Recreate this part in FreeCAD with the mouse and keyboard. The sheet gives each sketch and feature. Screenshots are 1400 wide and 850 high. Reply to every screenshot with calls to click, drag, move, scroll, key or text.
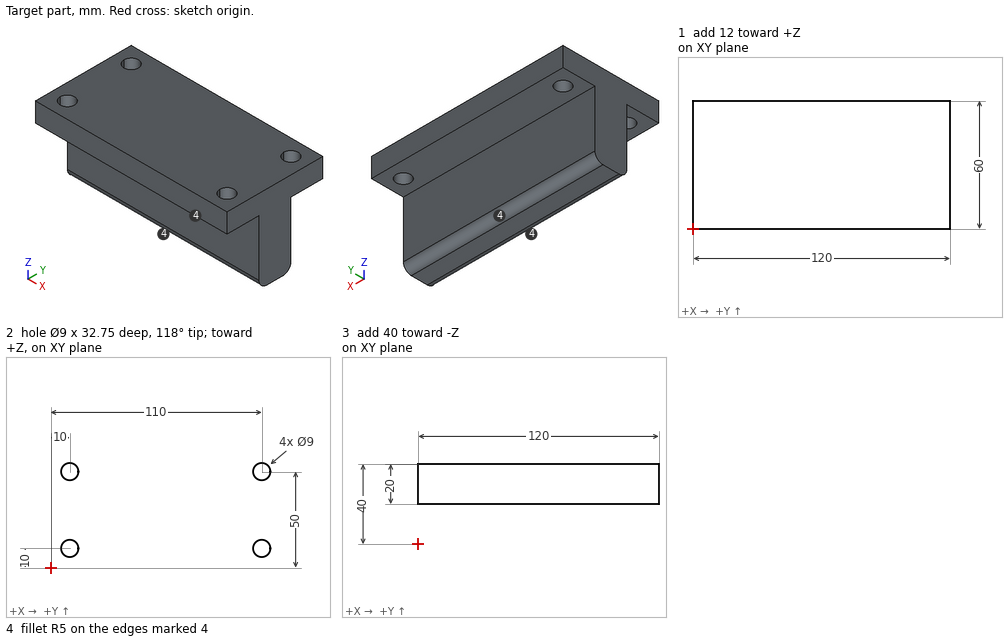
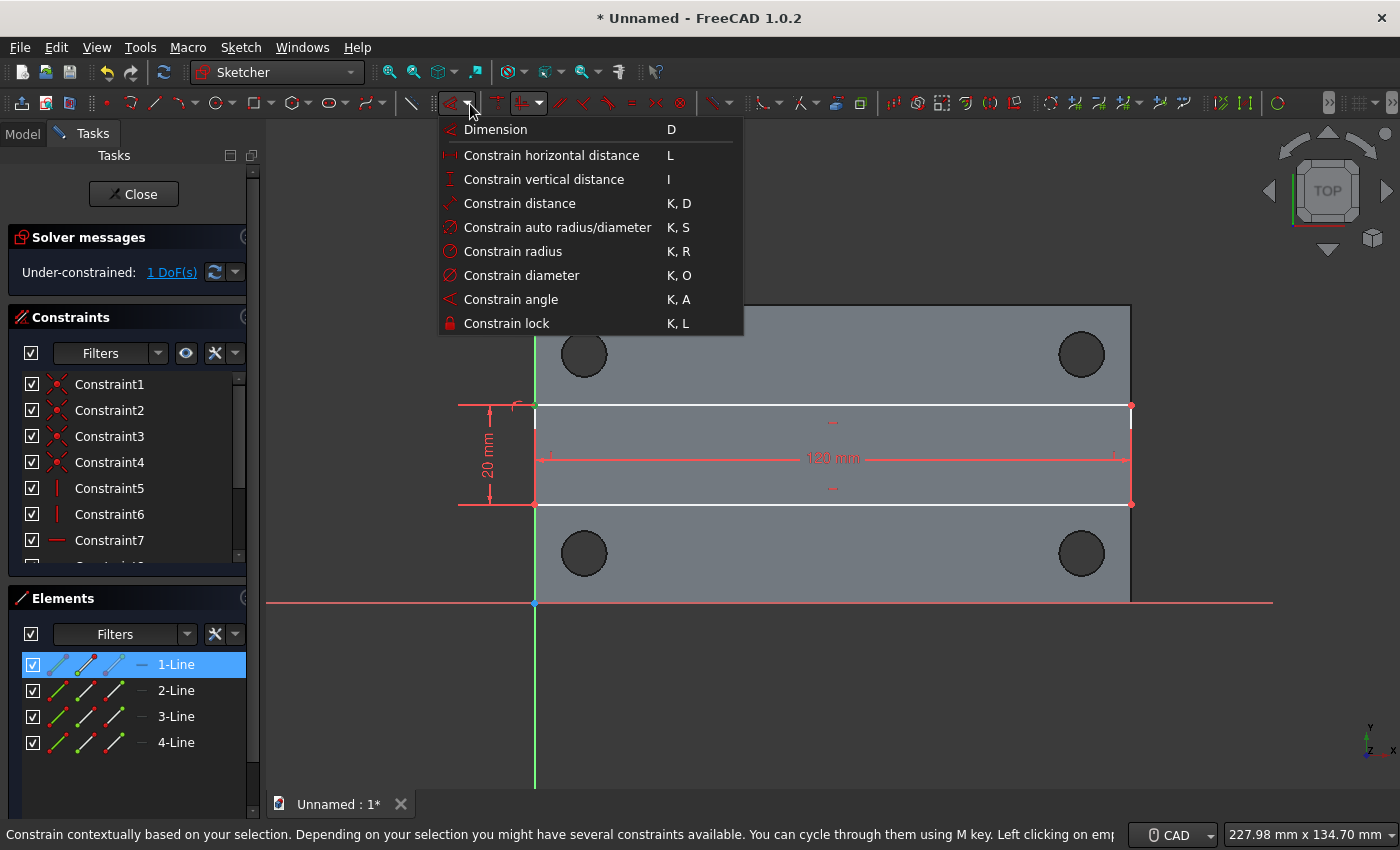
click(591, 179)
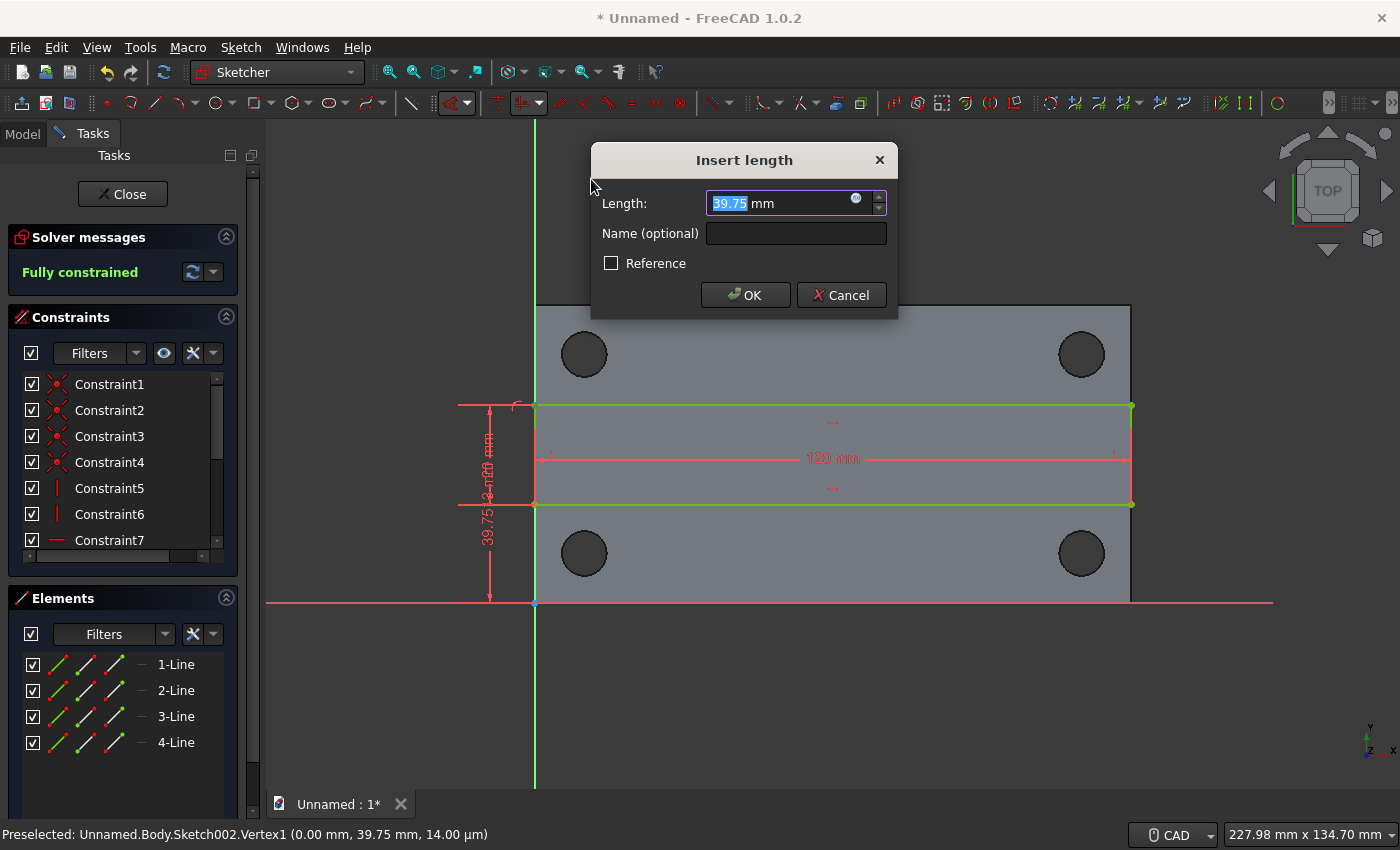
text(40)
key(Return)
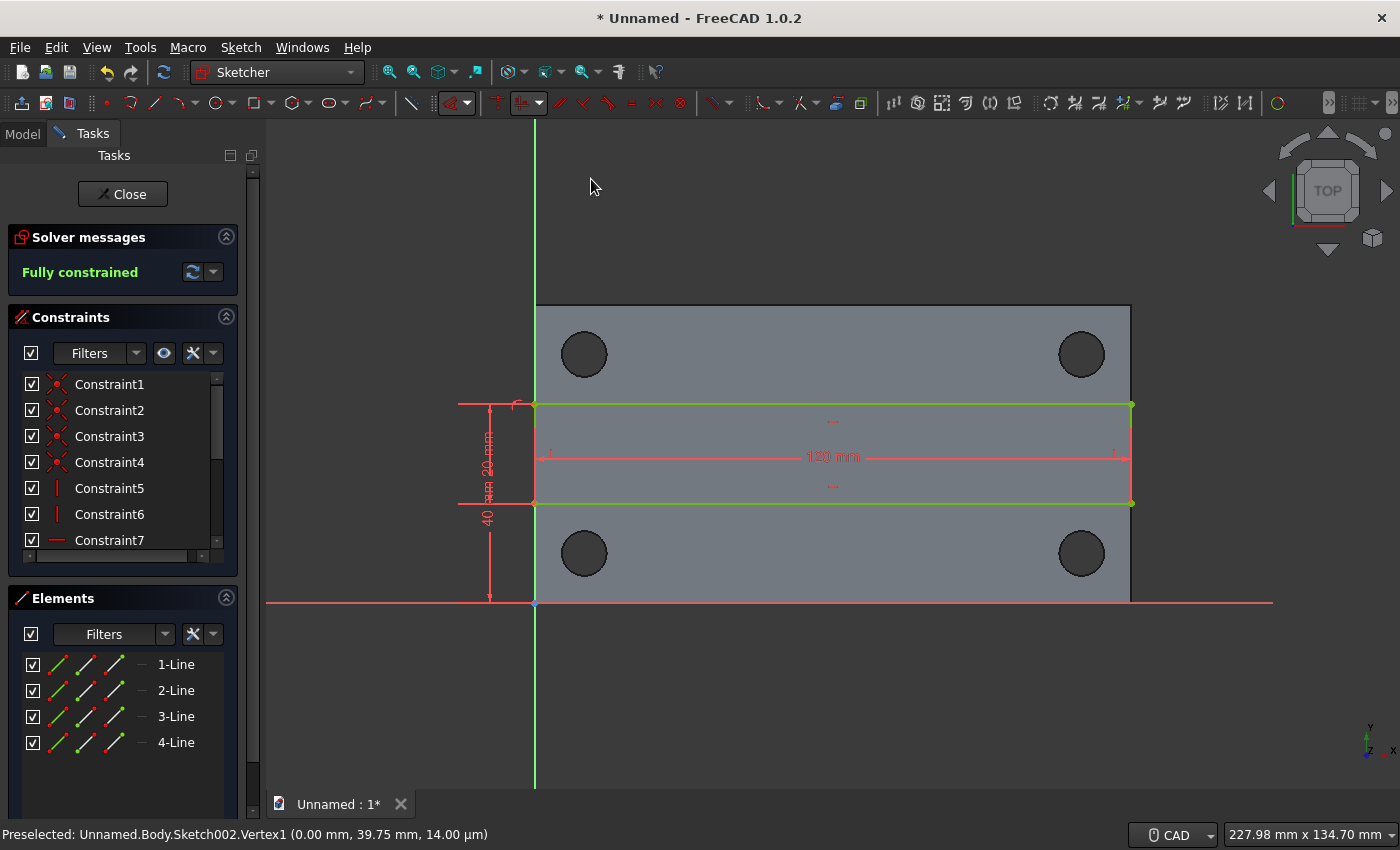
click(123, 194)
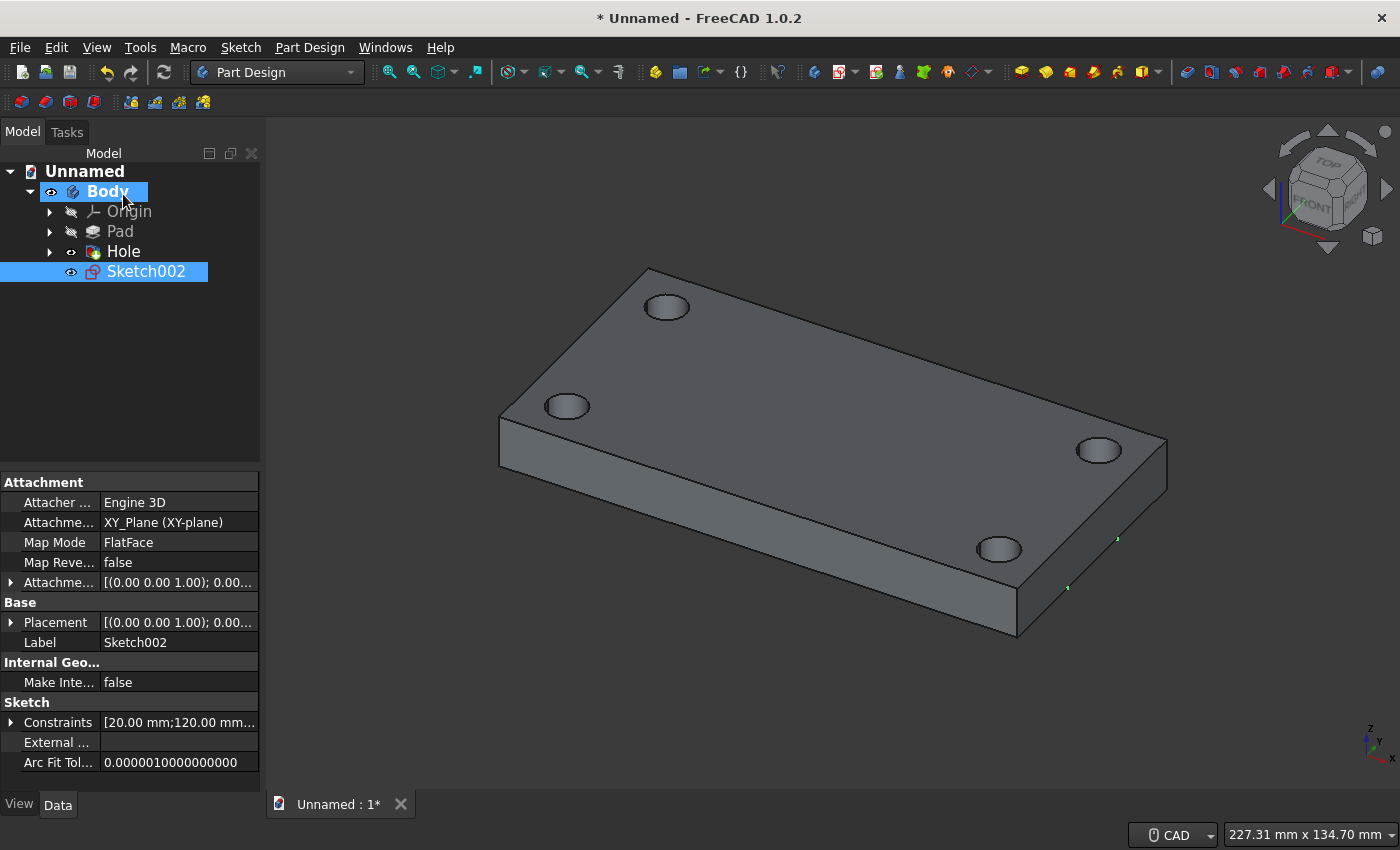
click(1022, 72)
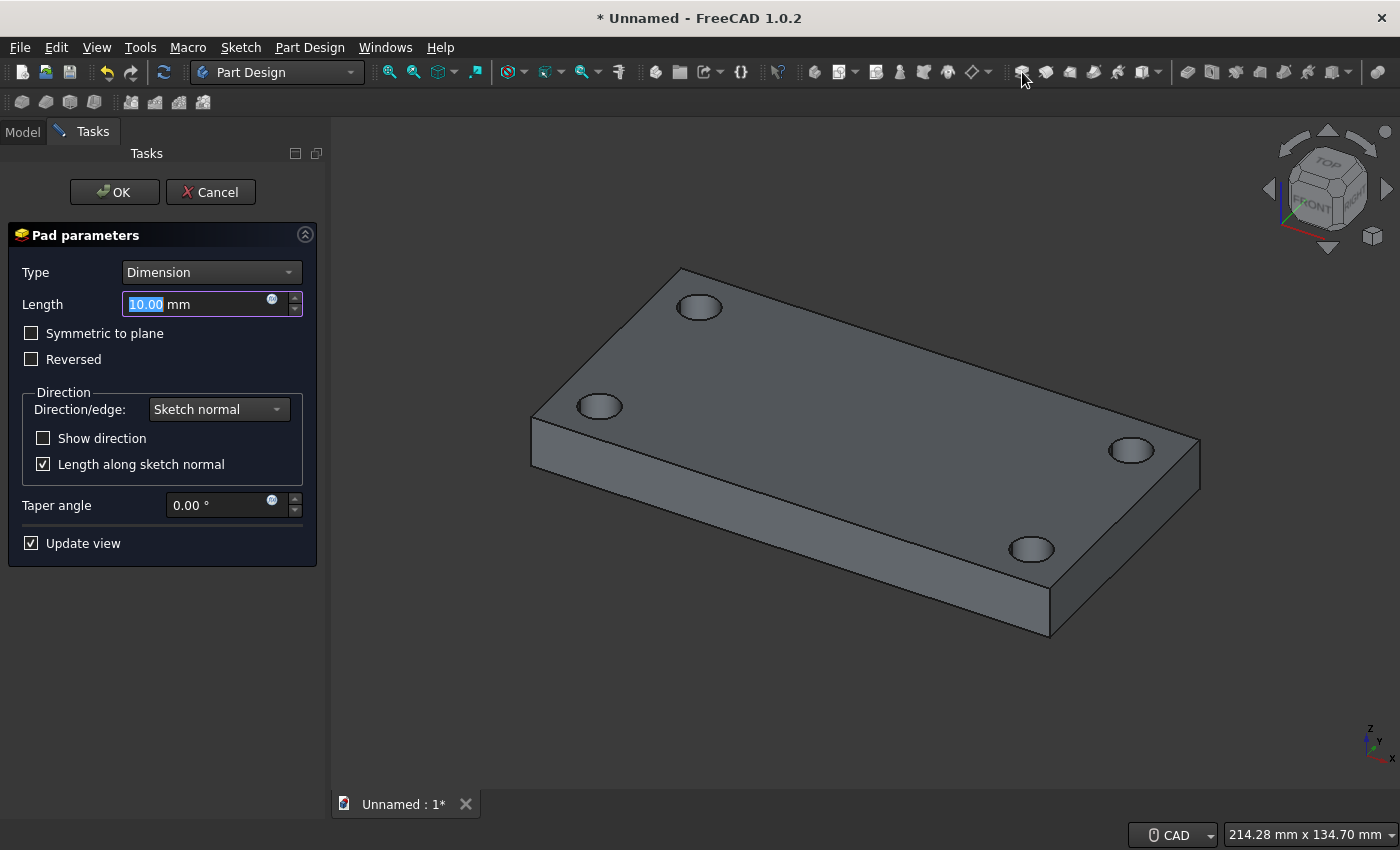
text(40)
key(Tab)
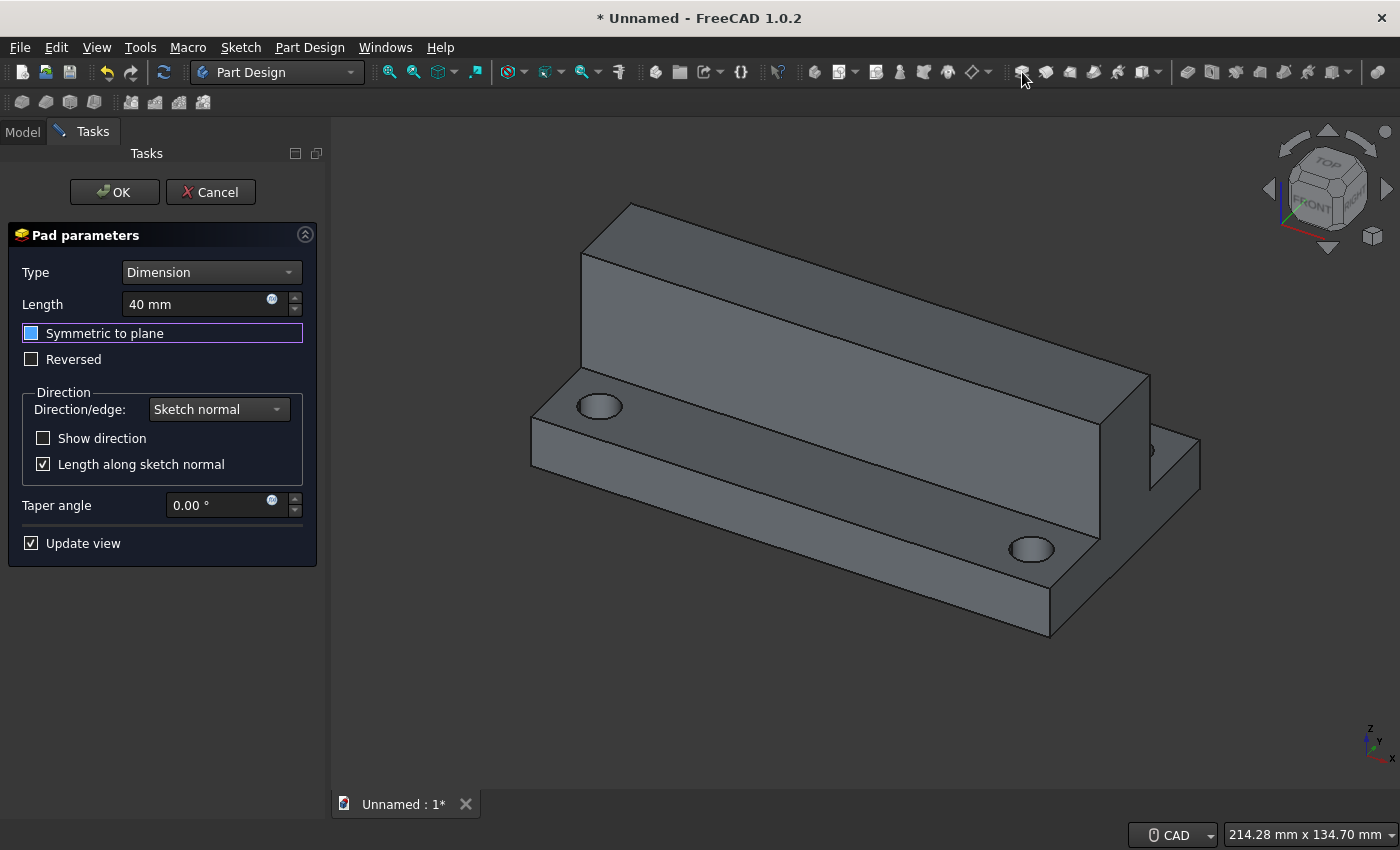
click(30, 359)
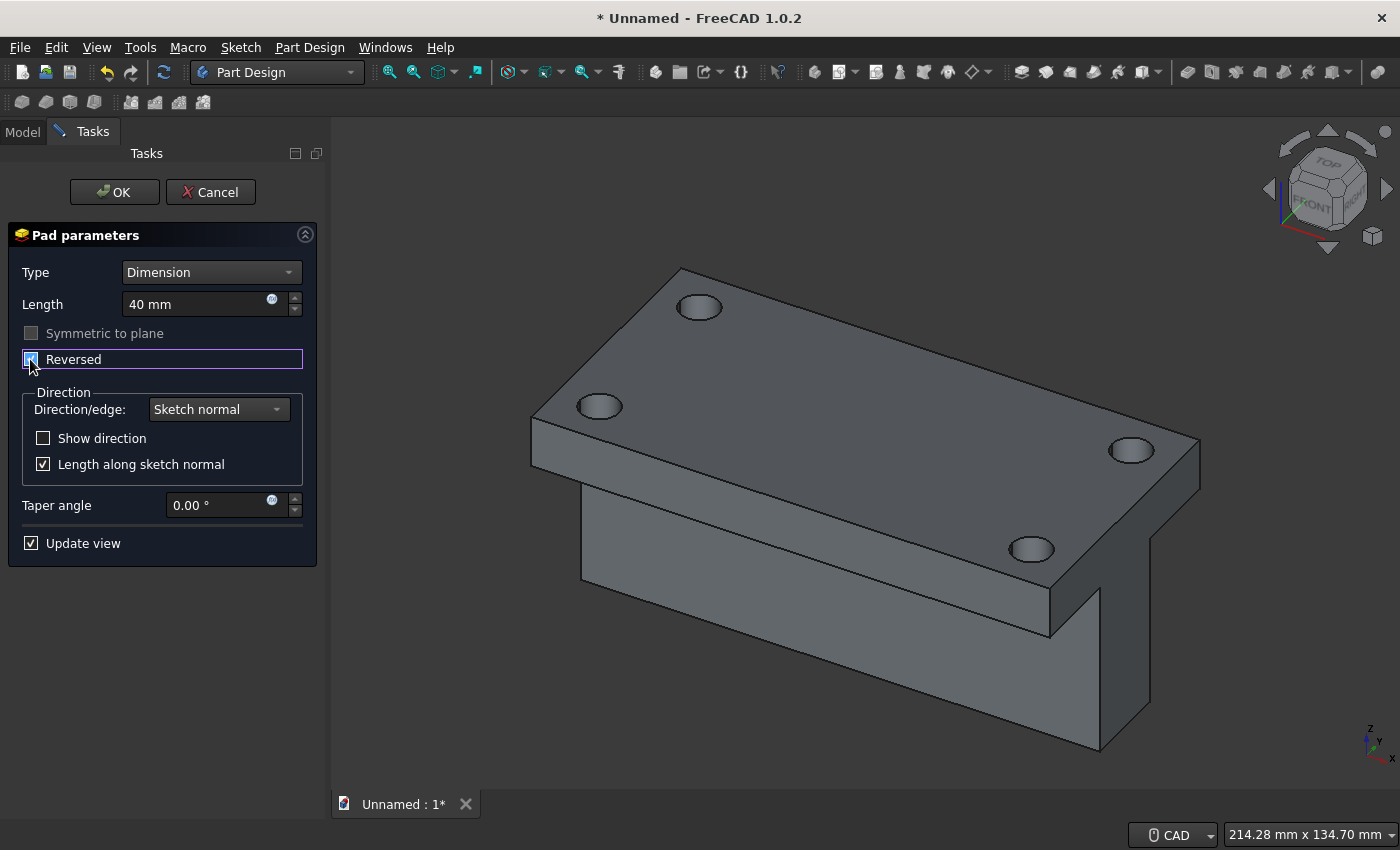
click(115, 192)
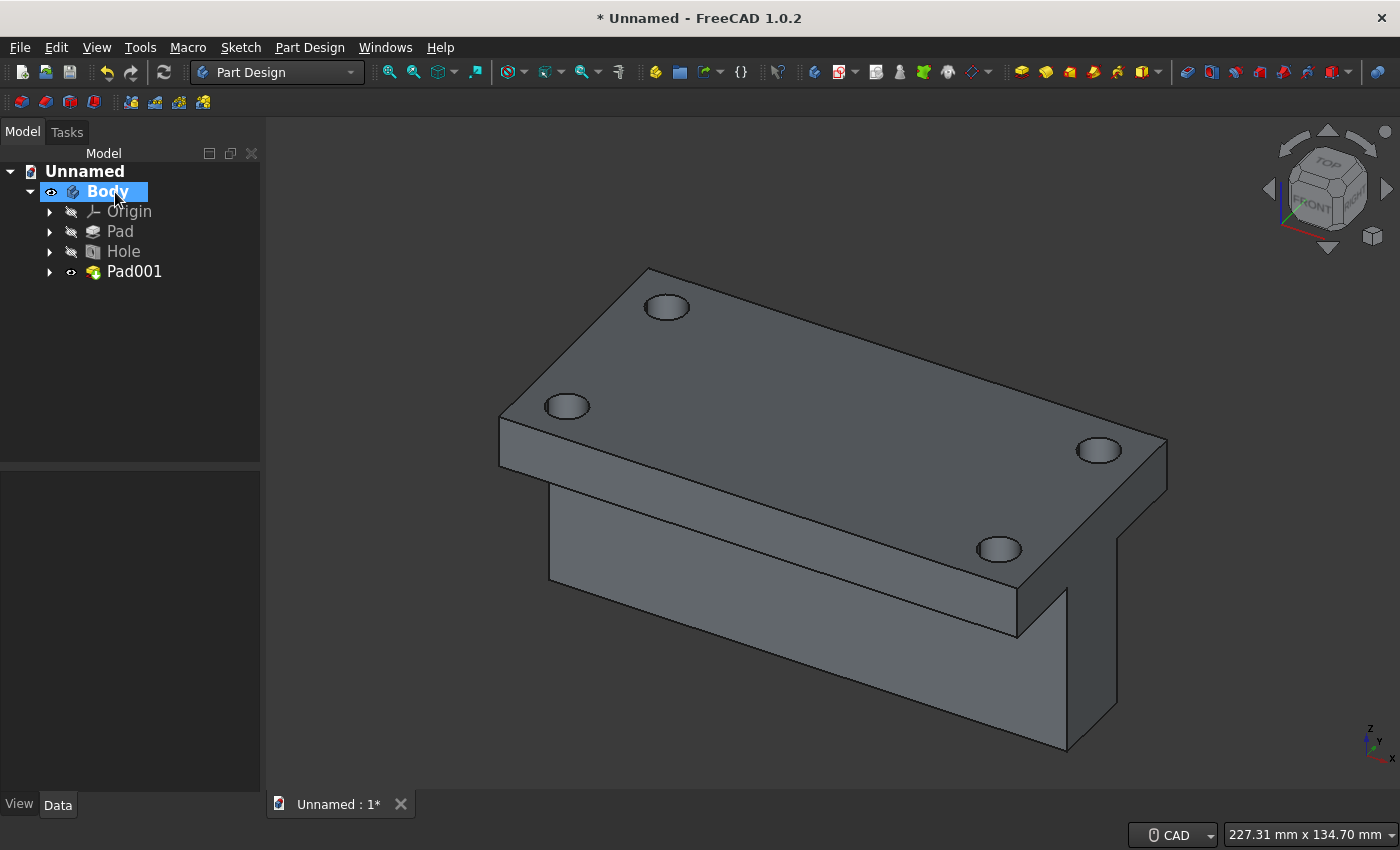
click(390, 72)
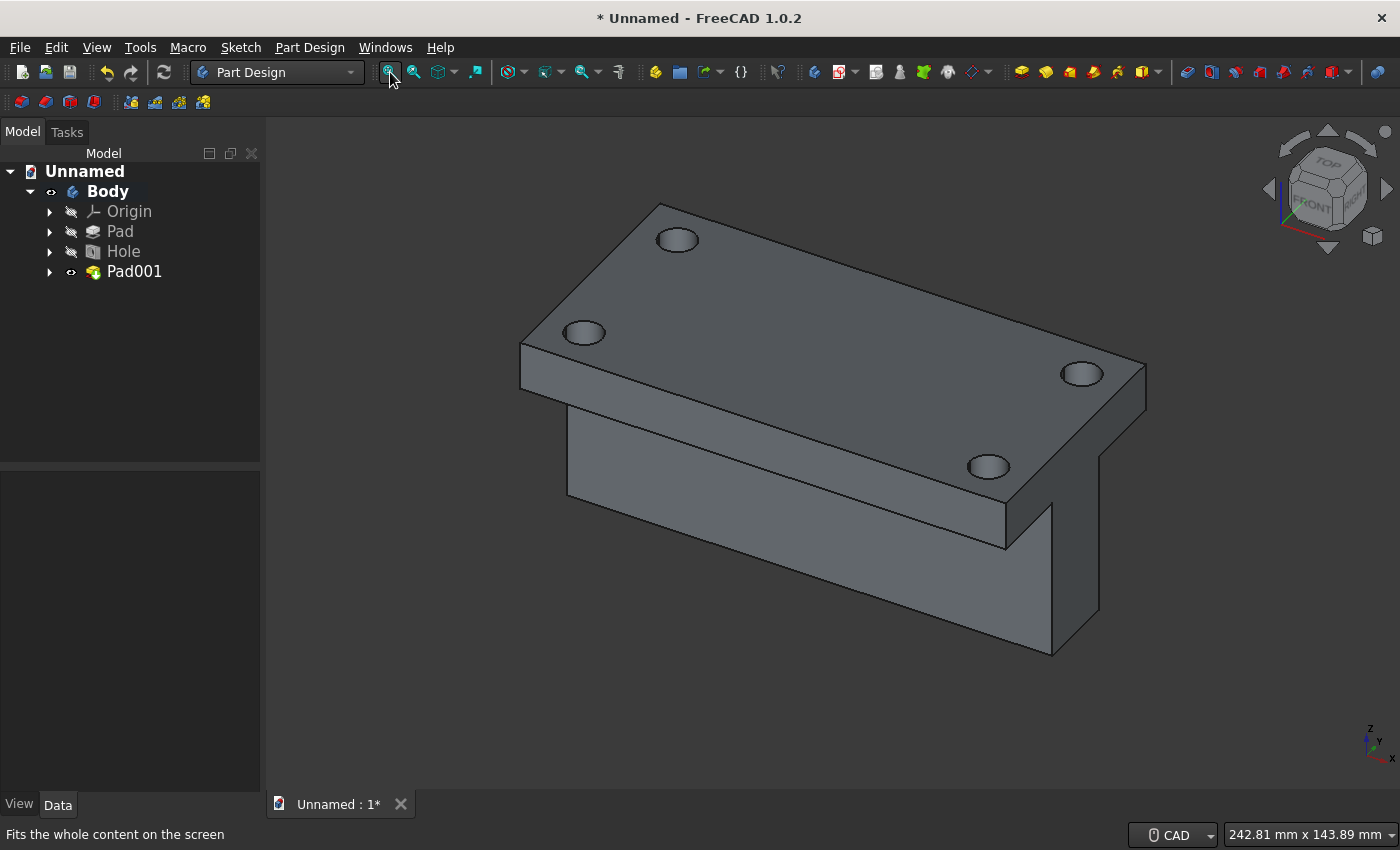
key(0)